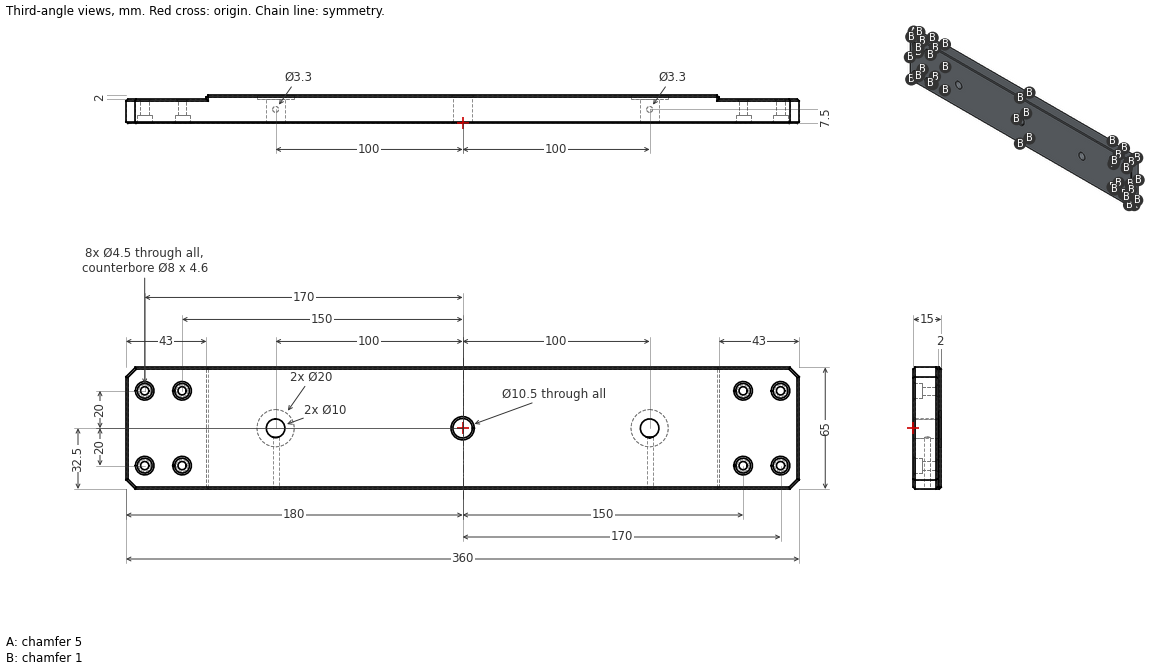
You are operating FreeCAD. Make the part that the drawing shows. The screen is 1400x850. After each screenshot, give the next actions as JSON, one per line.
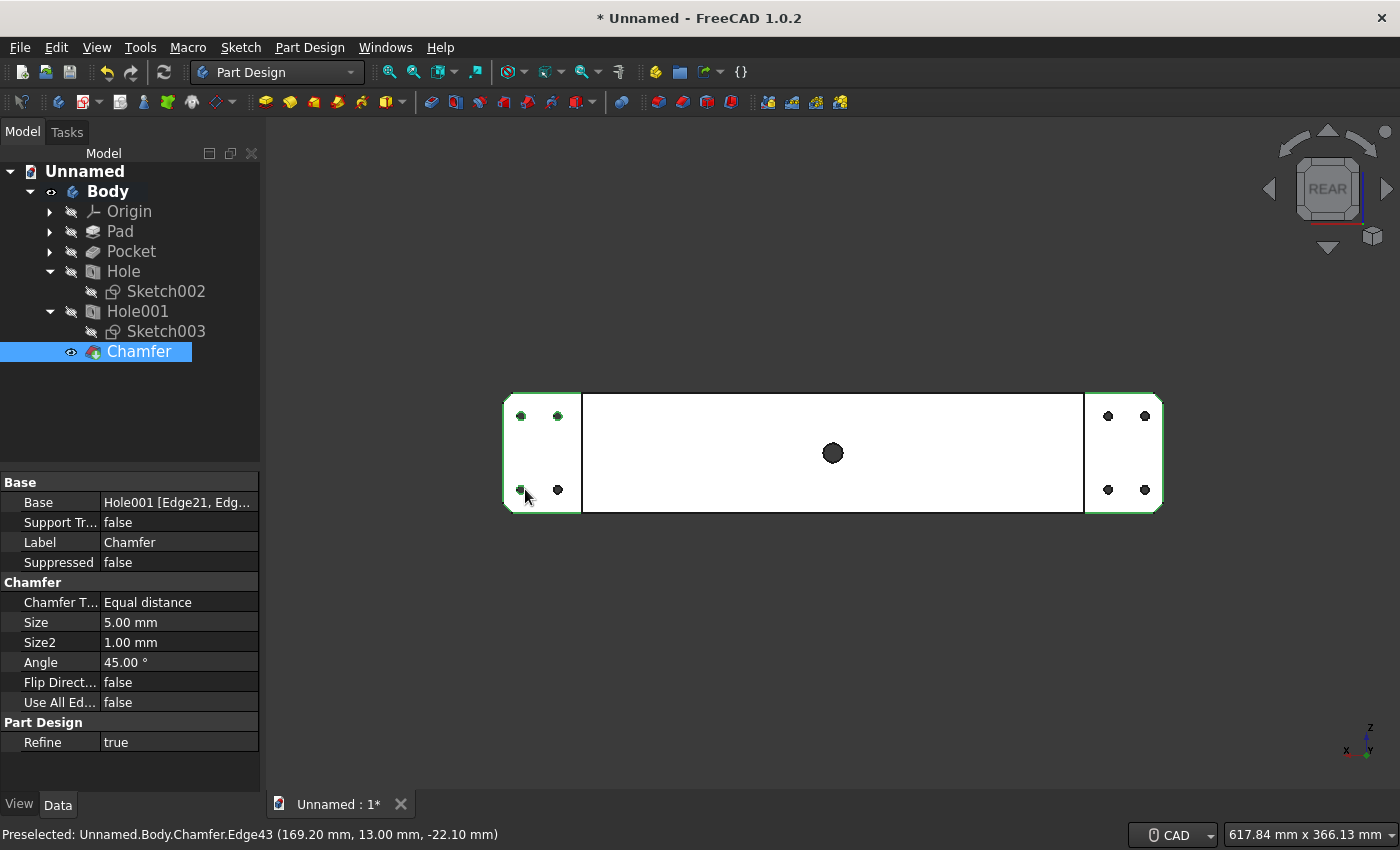
{"action": "left_click", "coordinate": [562, 489], "text": "ctrl"}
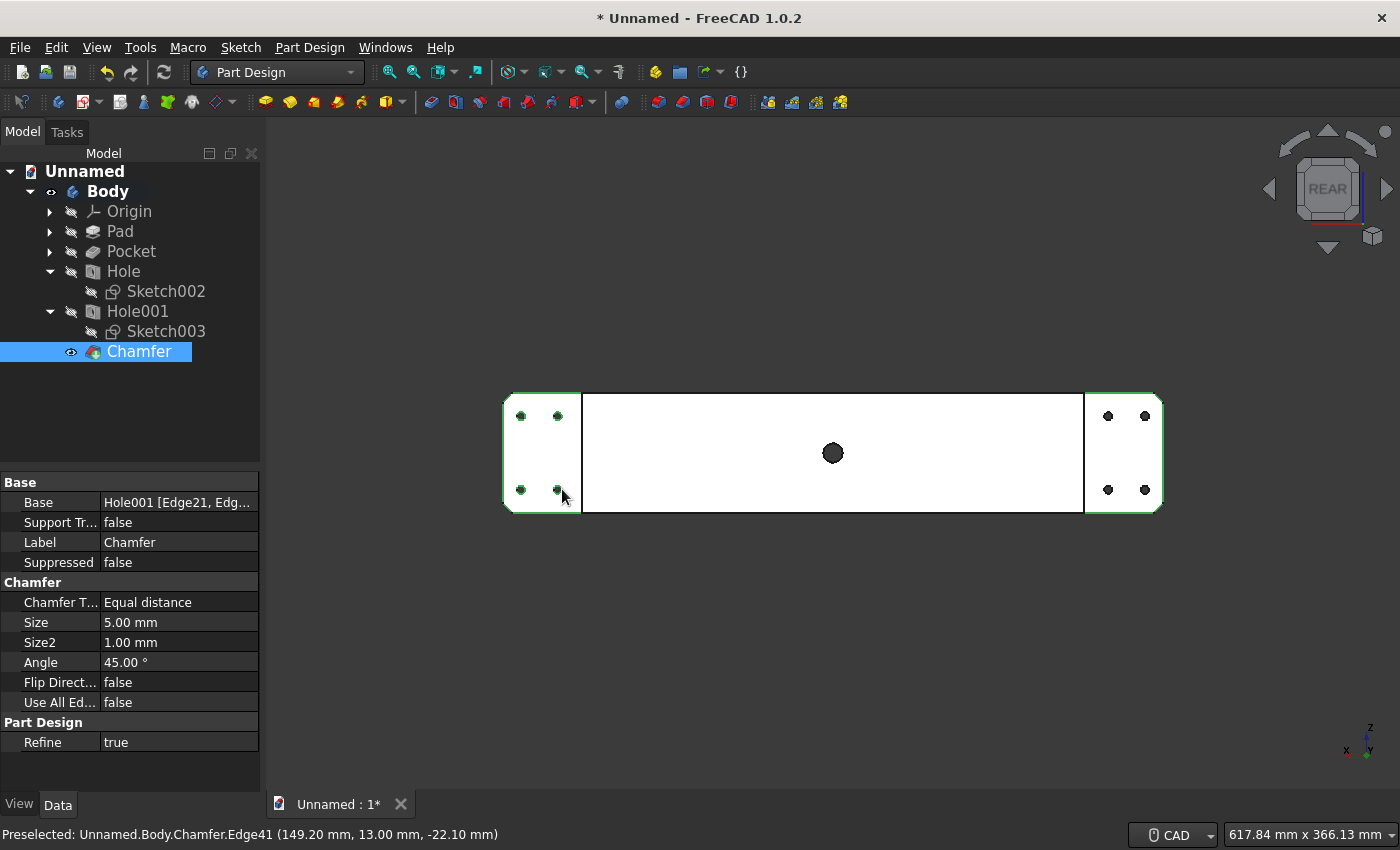
{"action": "left_click", "coordinate": [1112, 489], "text": "ctrl"}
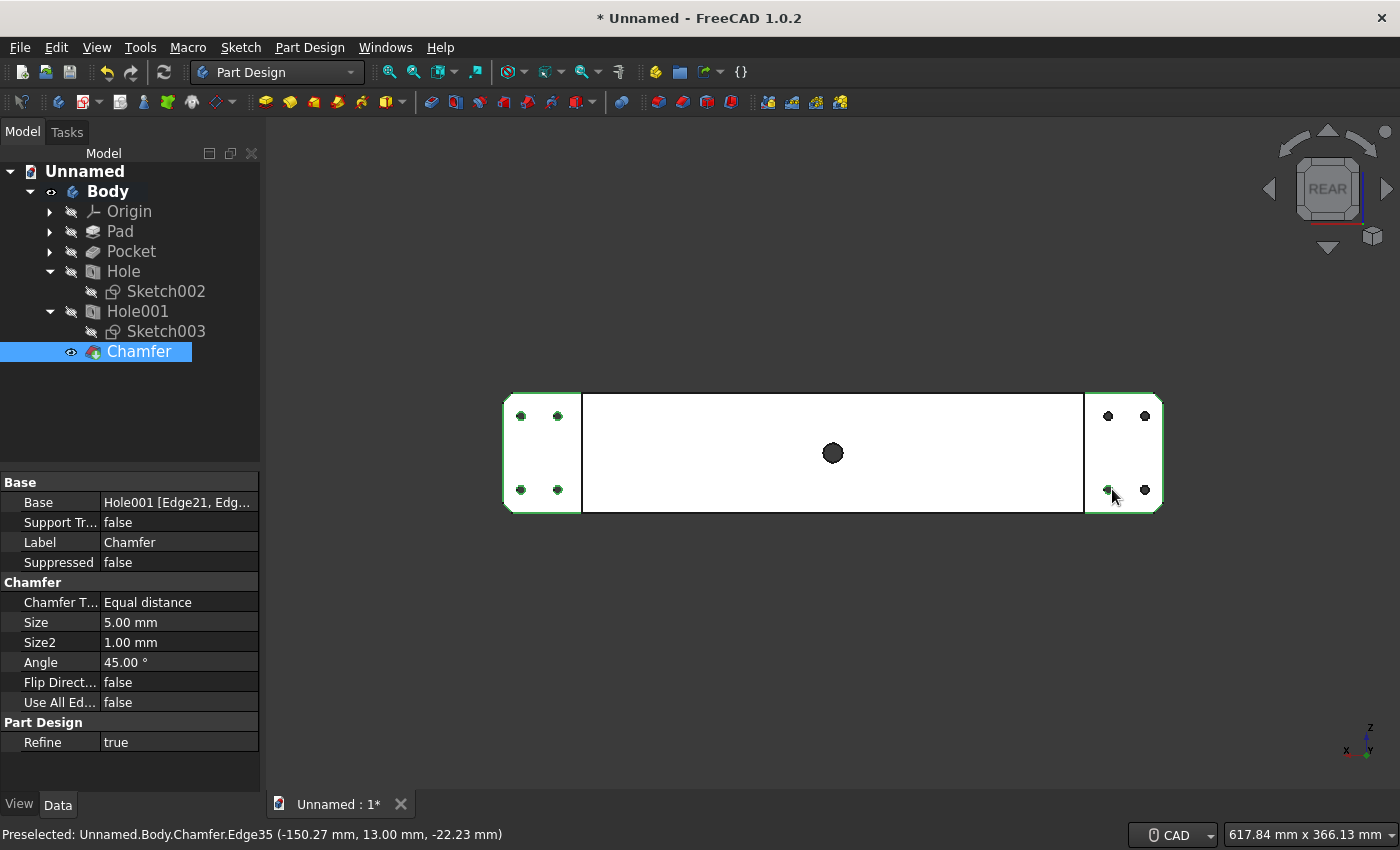
{"action": "left_click", "coordinate": [1149, 489], "text": "ctrl"}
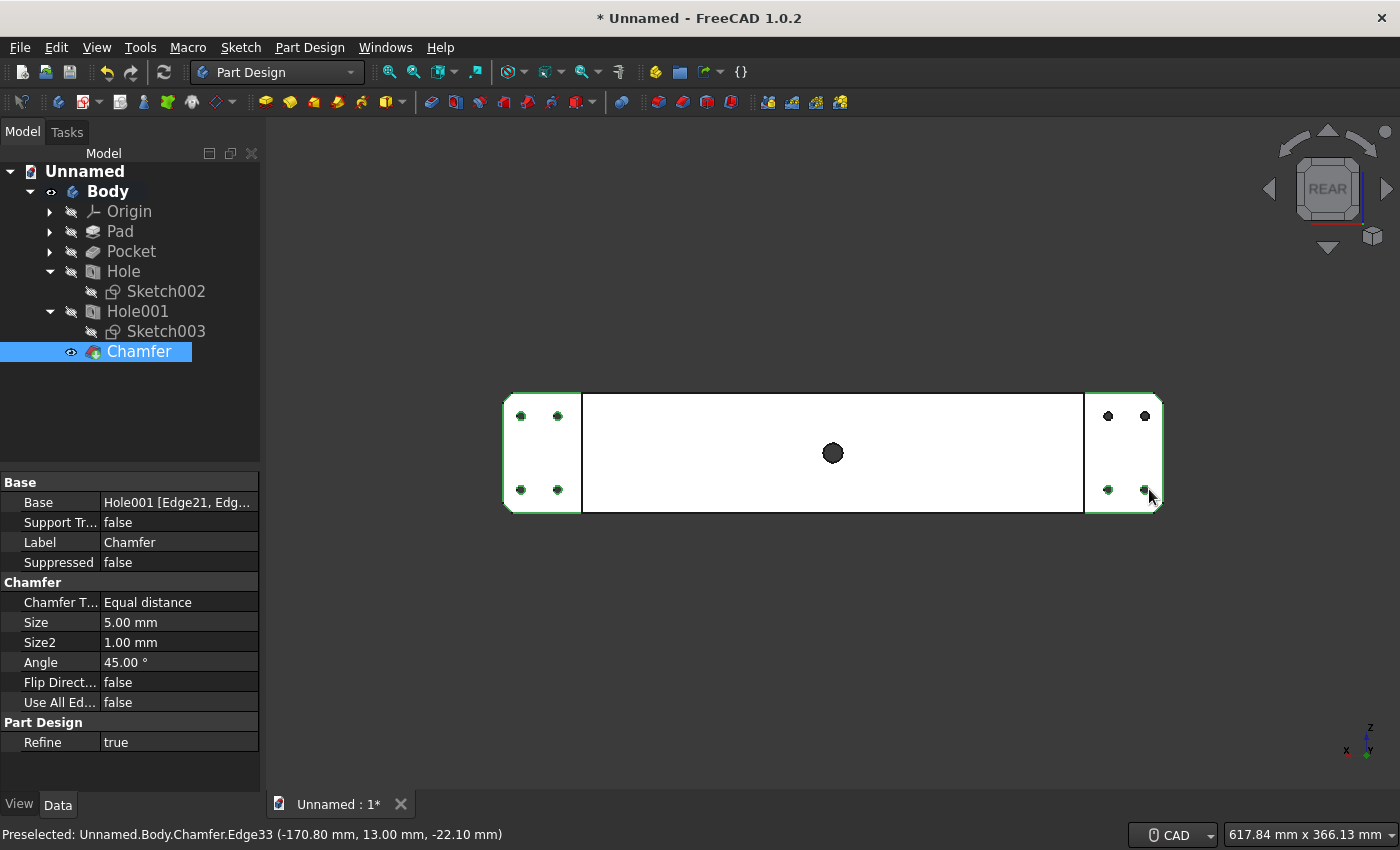
{"action": "left_click", "coordinate": [1112, 415], "text": "ctrl"}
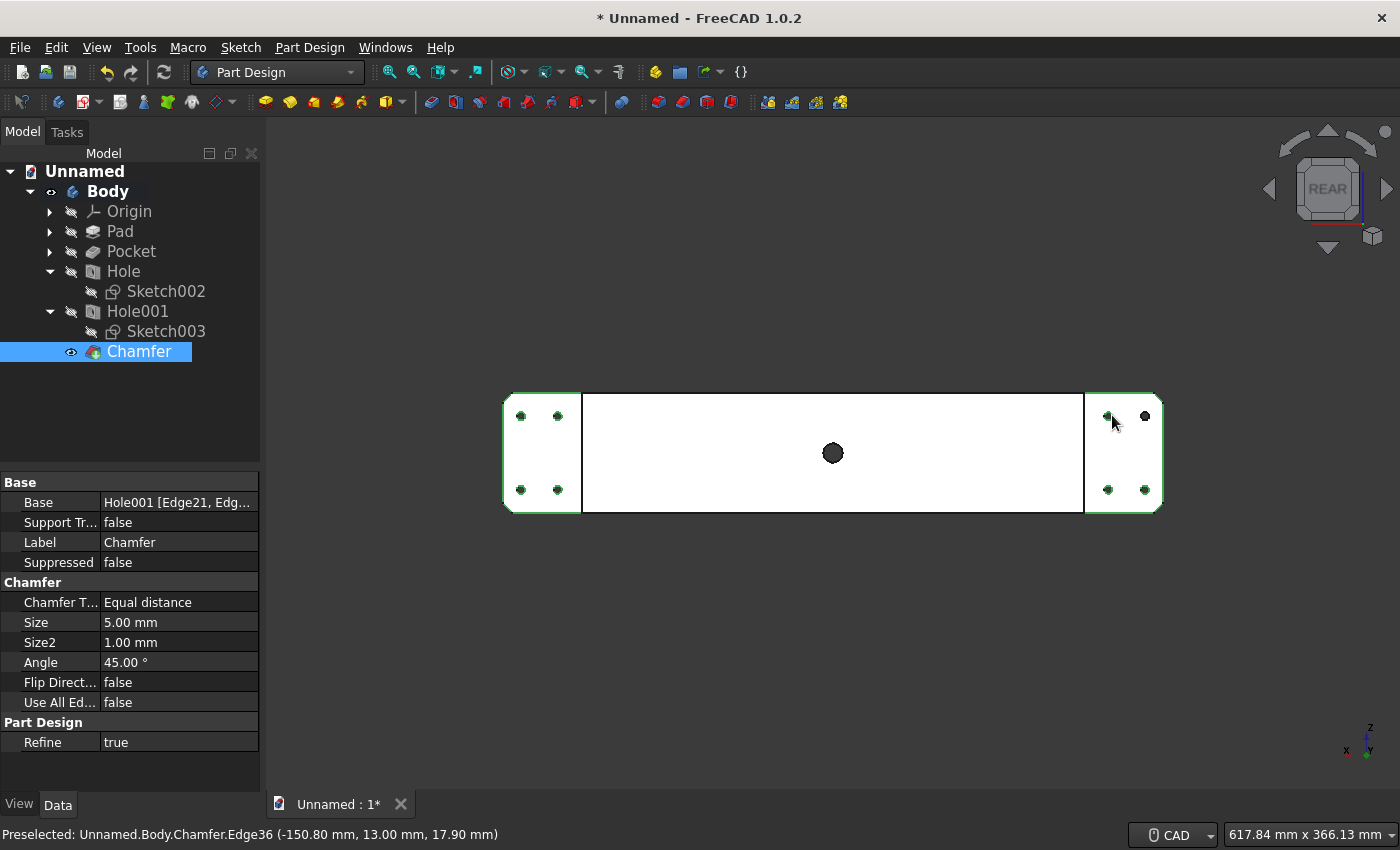
{"action": "left_click", "coordinate": [1149, 415], "text": "ctrl"}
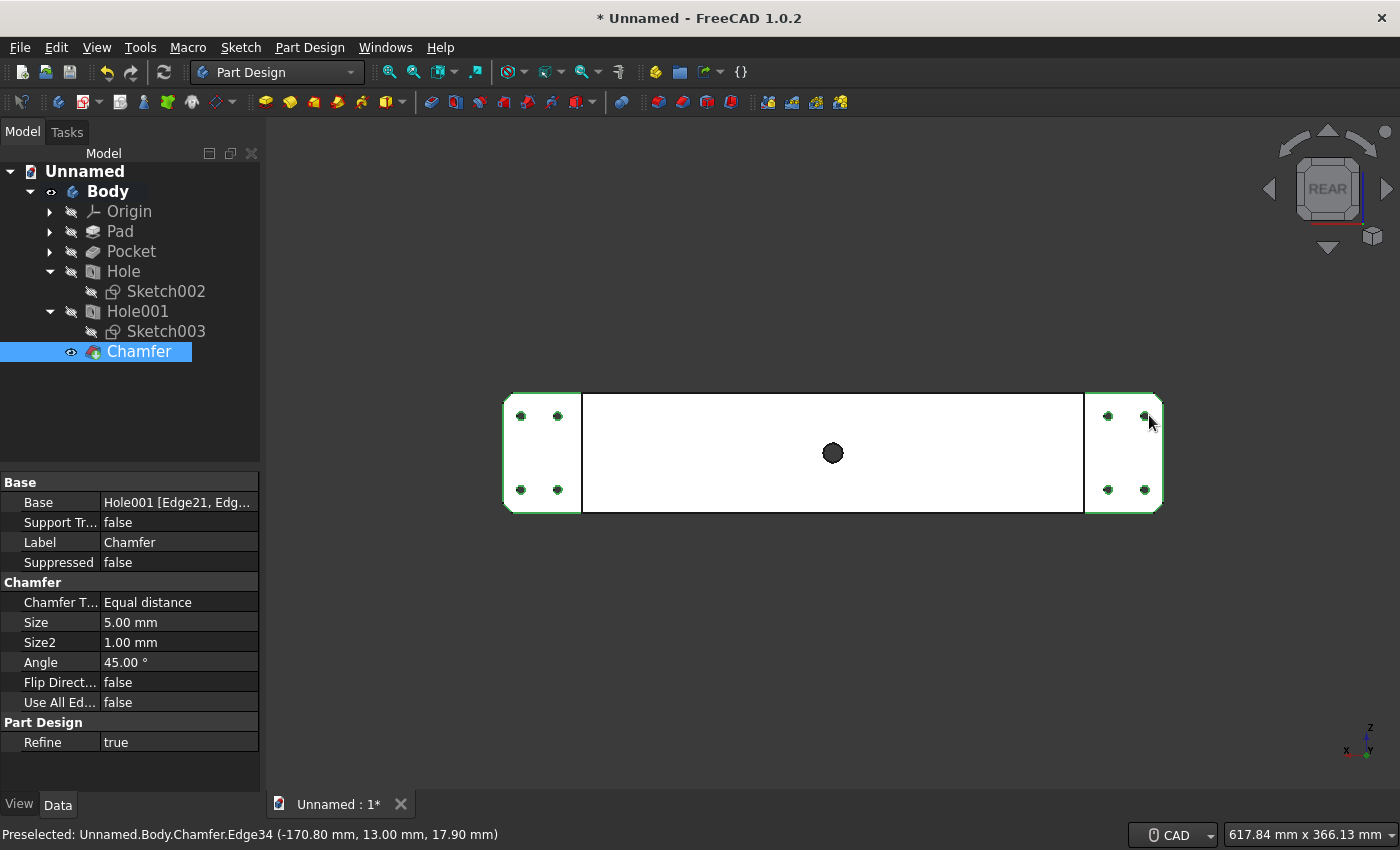
{"action": "scroll", "coordinate": [1084, 512], "scroll_direction": "up", "scroll_amount": 12}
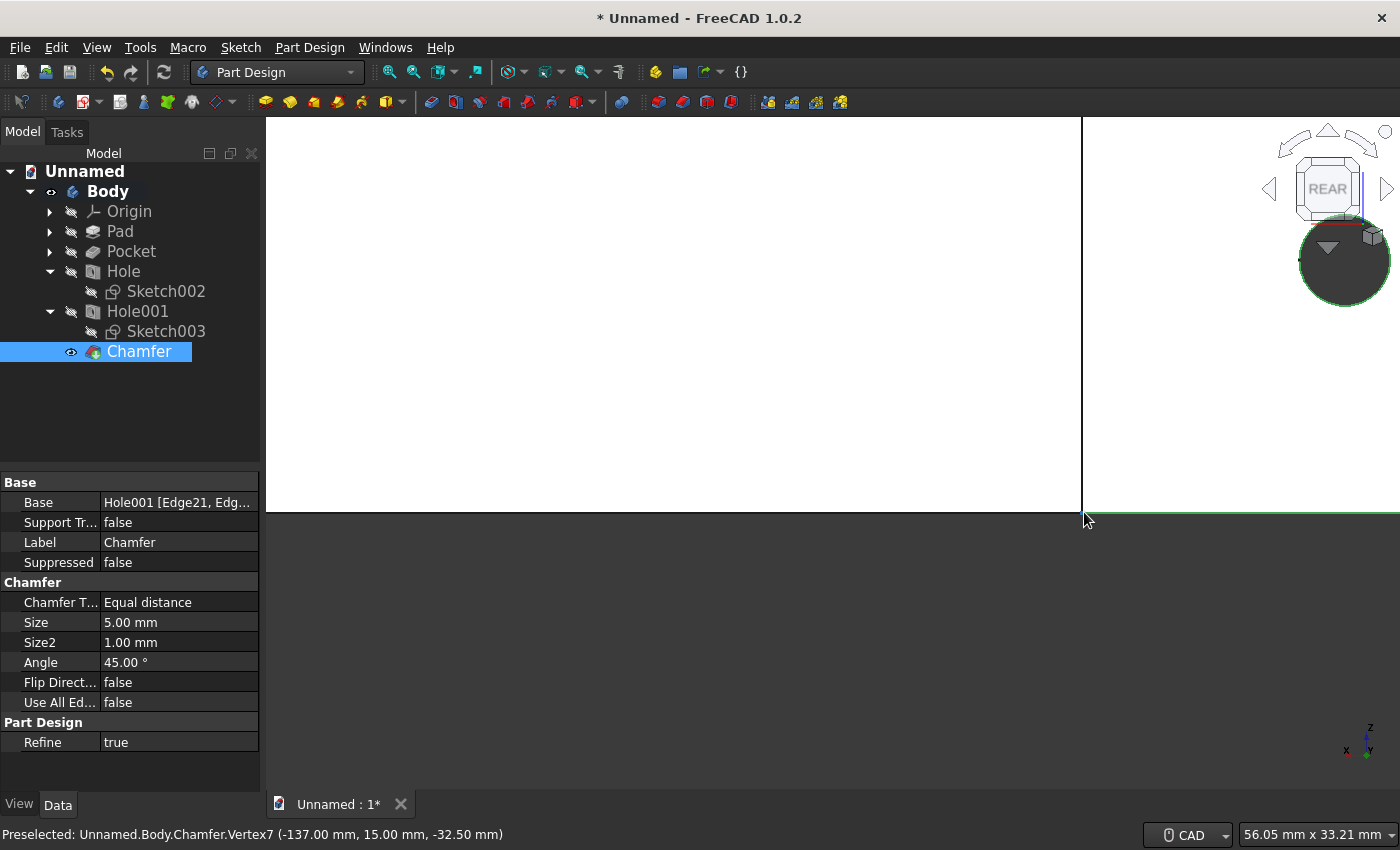
{"action": "left_click", "coordinate": [390, 72]}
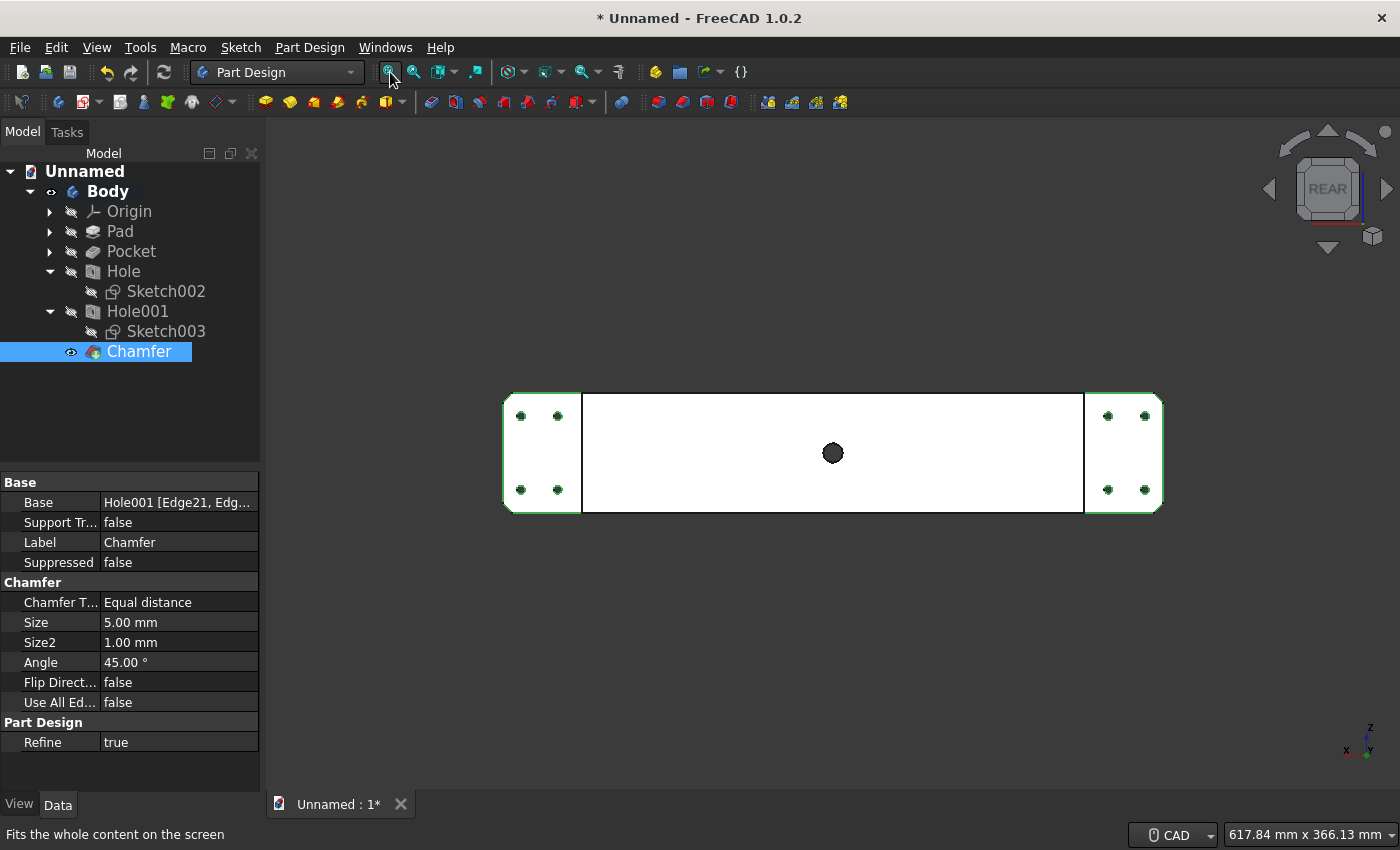
{"action": "key", "text": "6"}